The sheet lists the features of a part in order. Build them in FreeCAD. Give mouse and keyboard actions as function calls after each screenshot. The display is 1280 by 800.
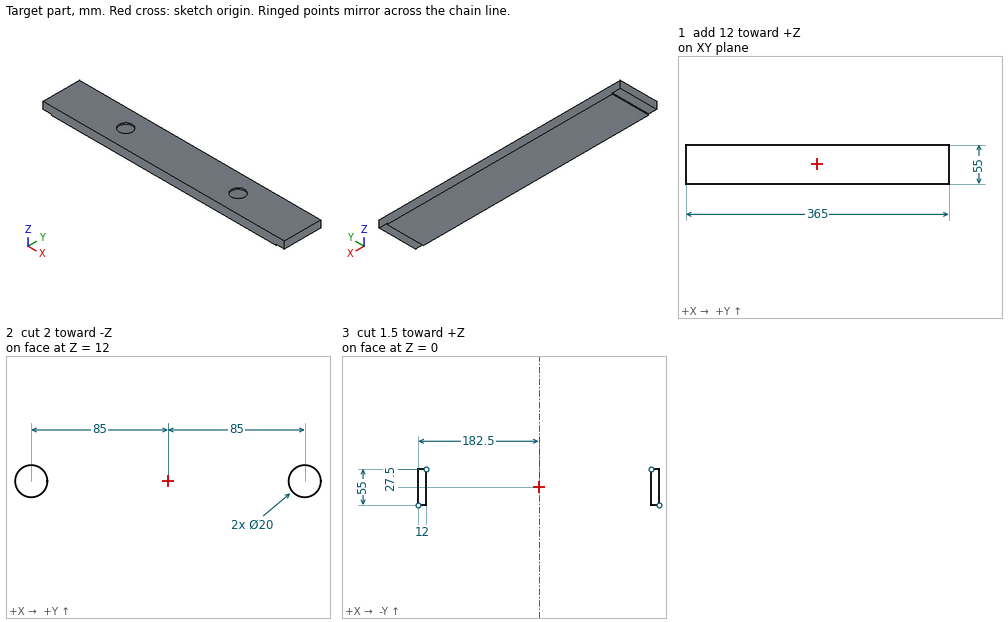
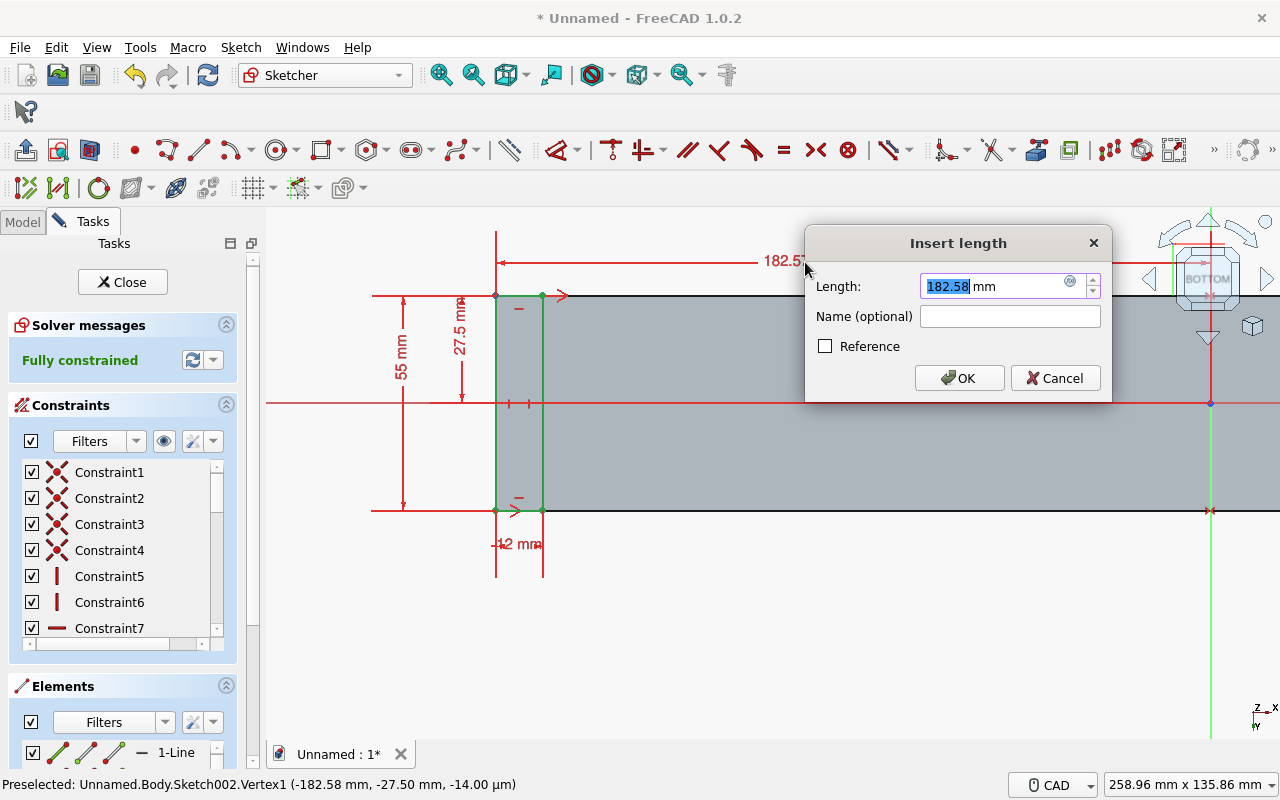
text(182.5)
key(Return)
key(Escape)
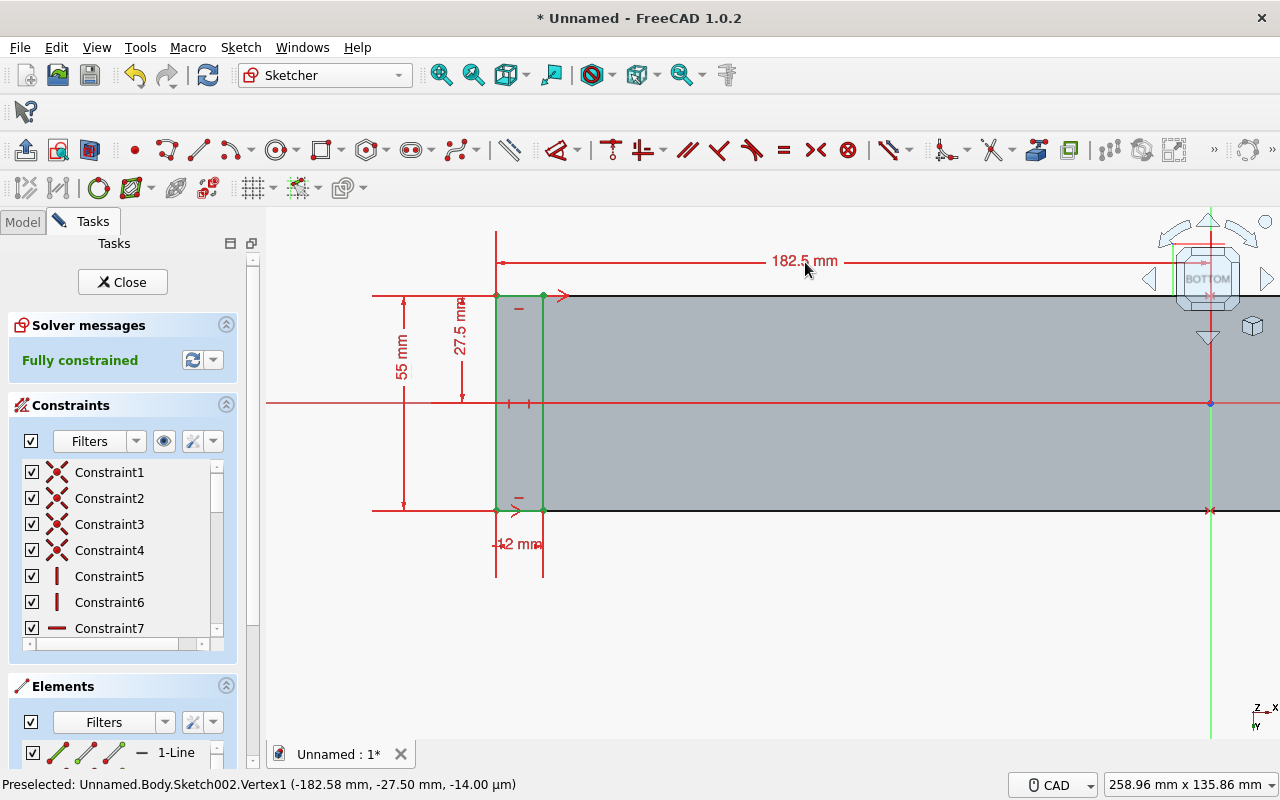
click(123, 282)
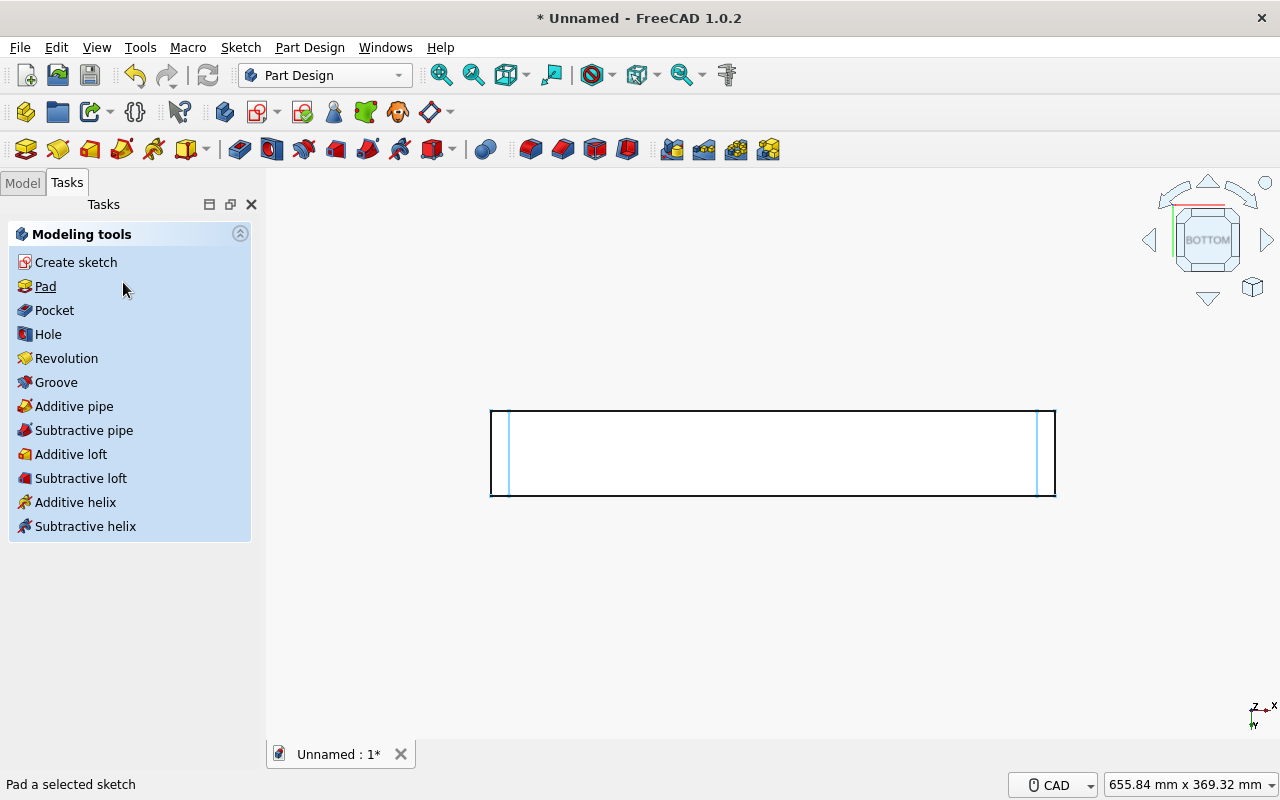
click(240, 150)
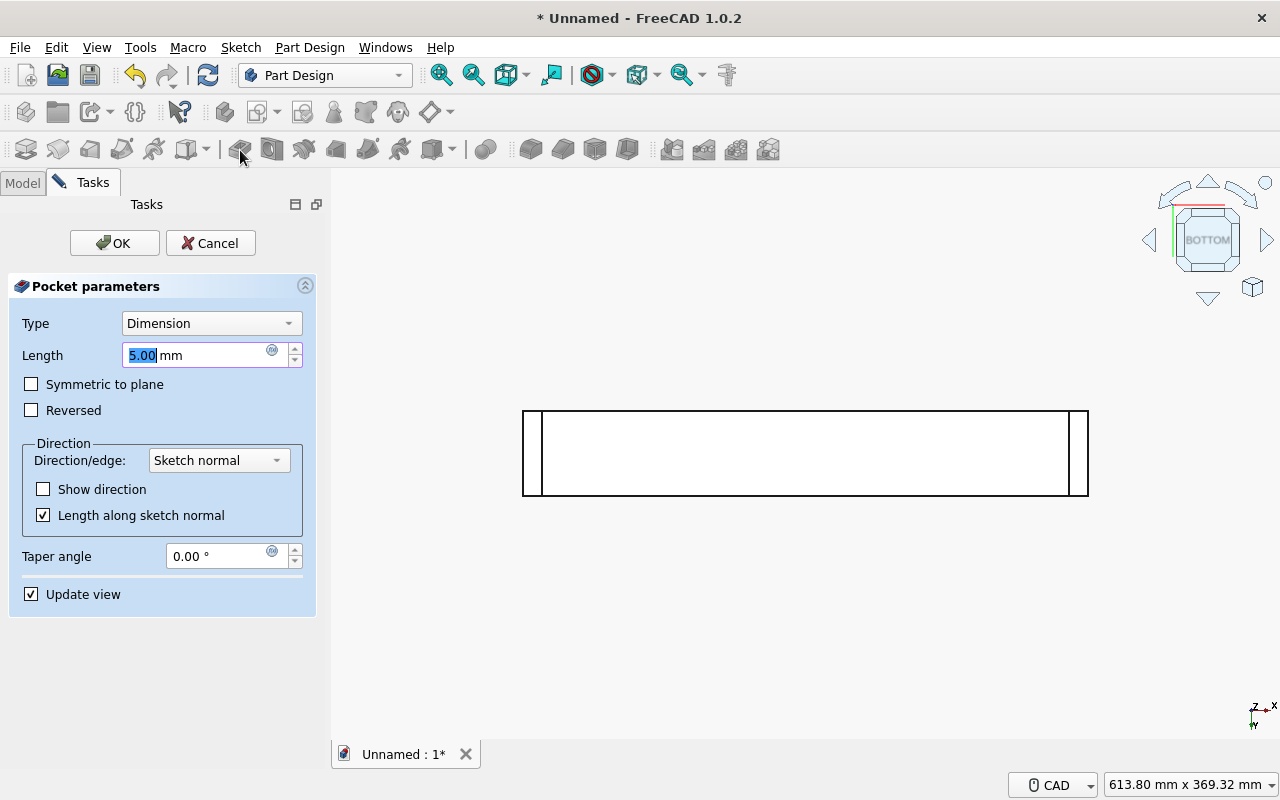
text(1.5)
key(Tab)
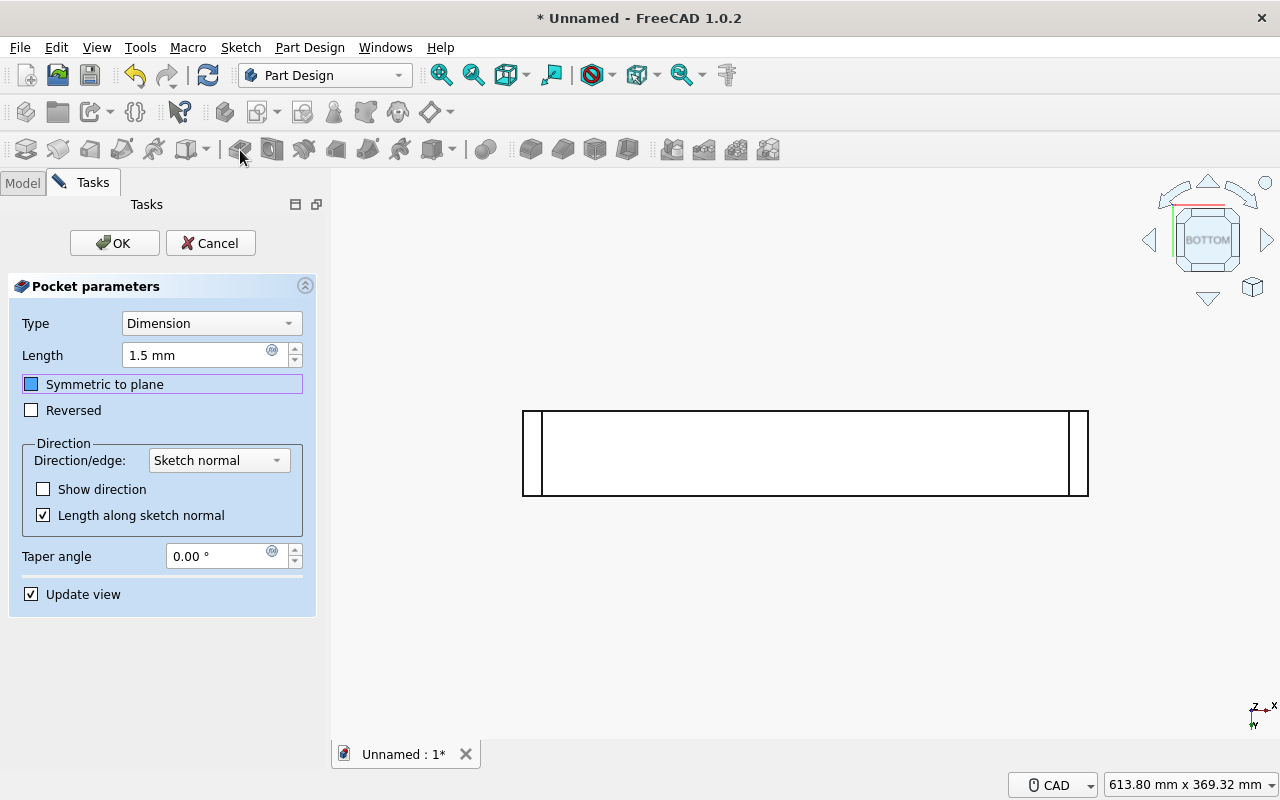
click(115, 243)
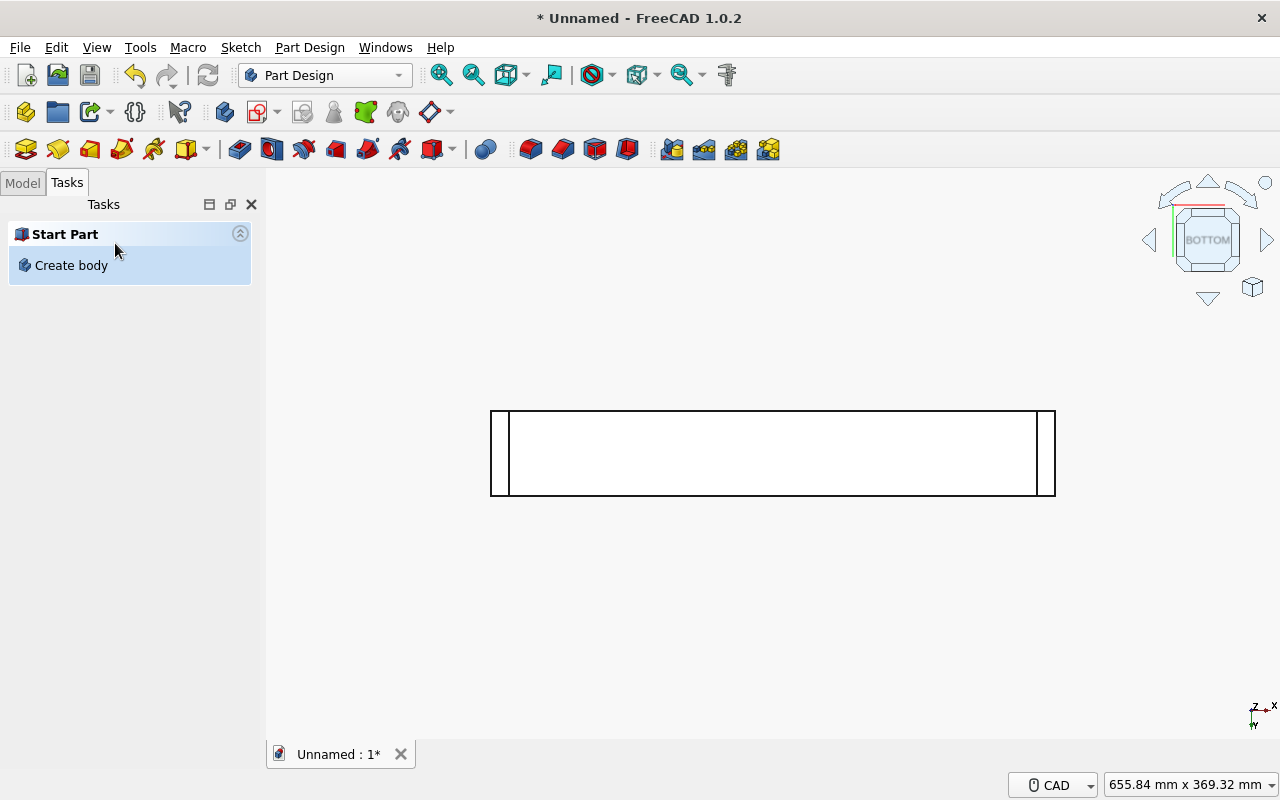
key(0)